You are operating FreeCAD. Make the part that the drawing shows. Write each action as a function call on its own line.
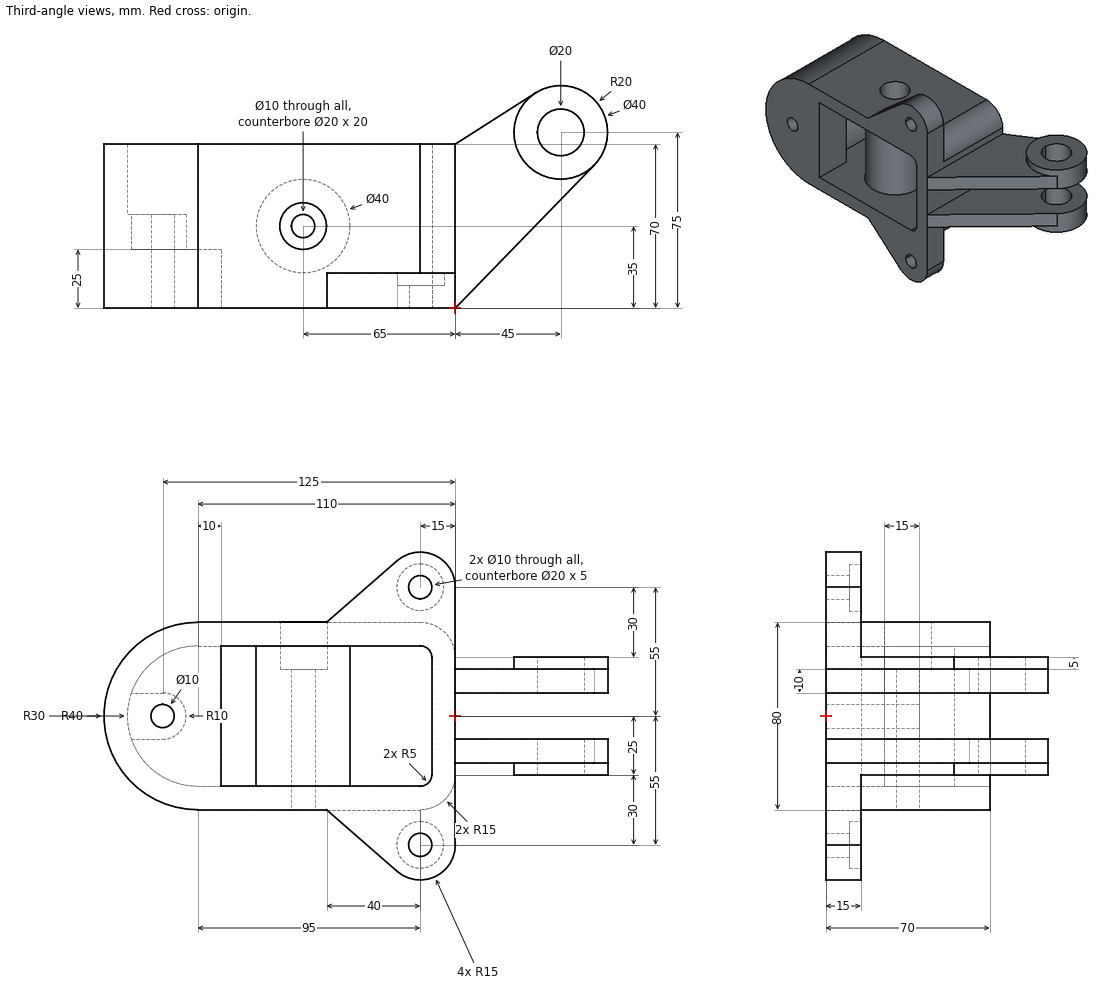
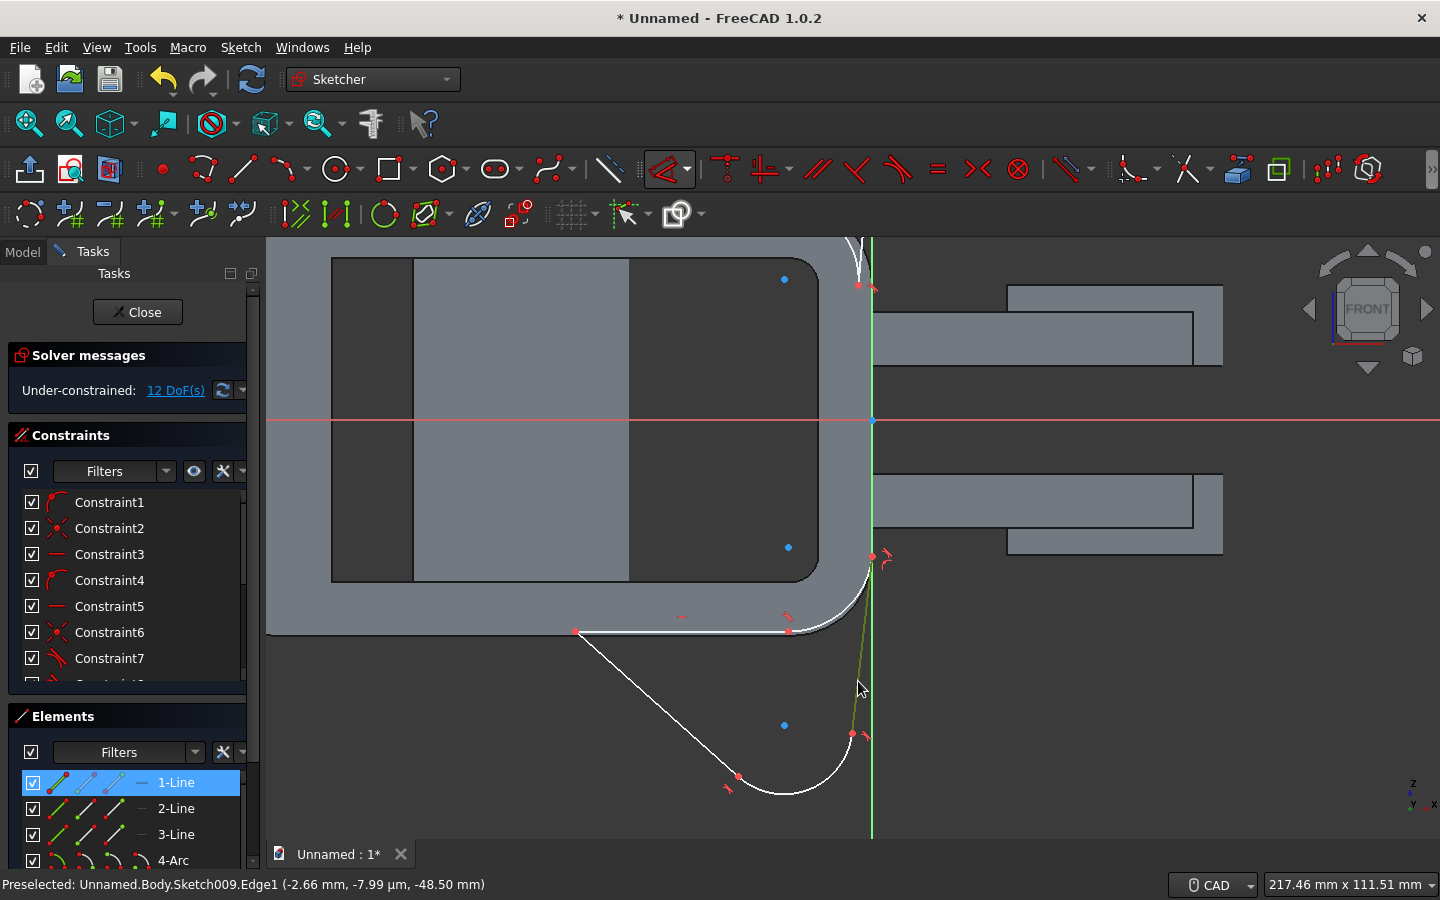
key(v)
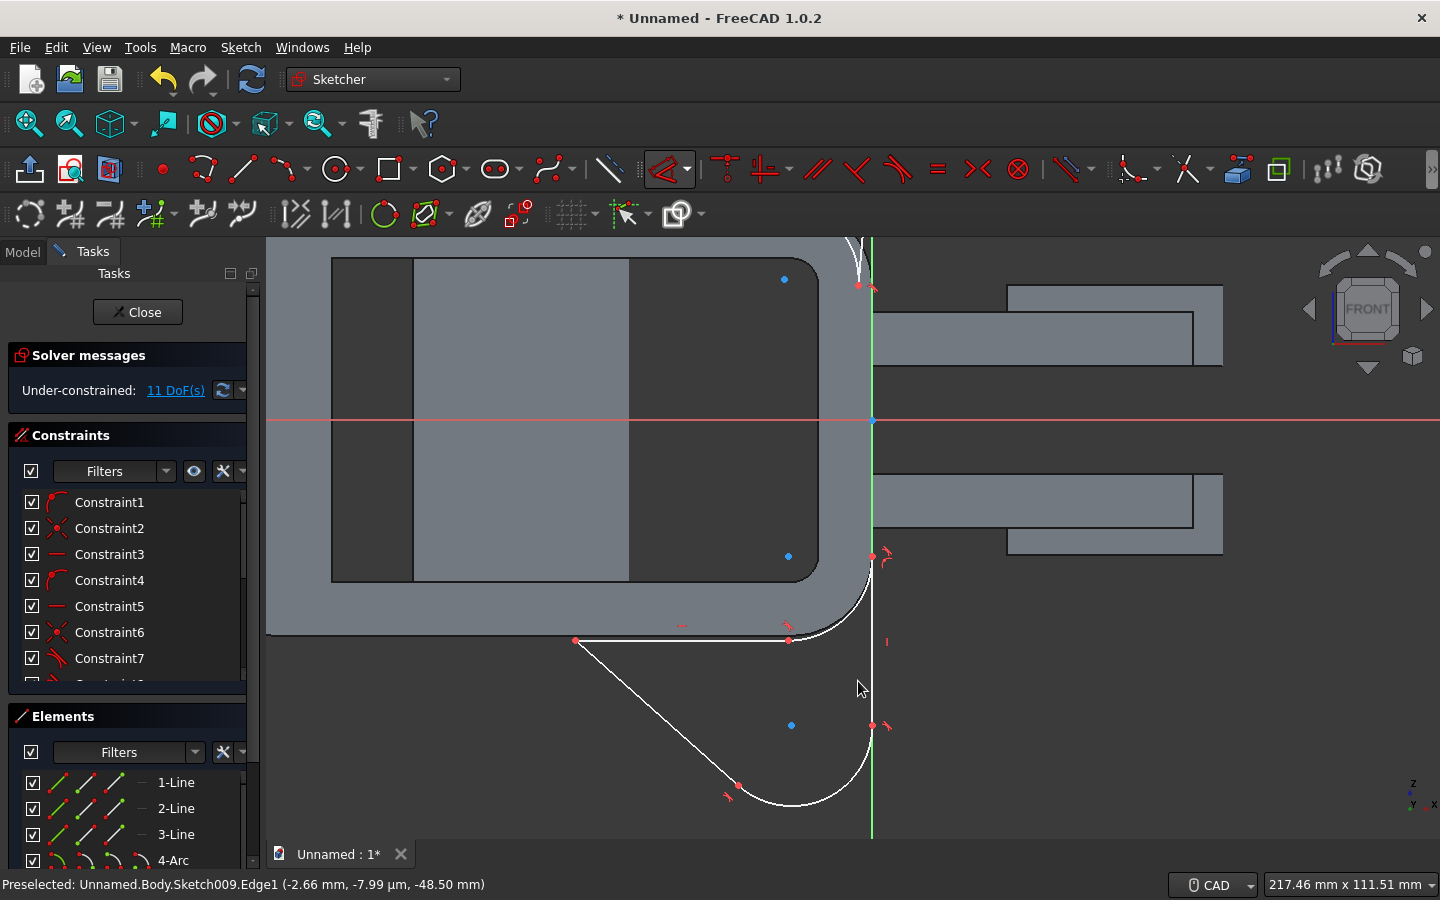
scroll(858, 681, down, 3)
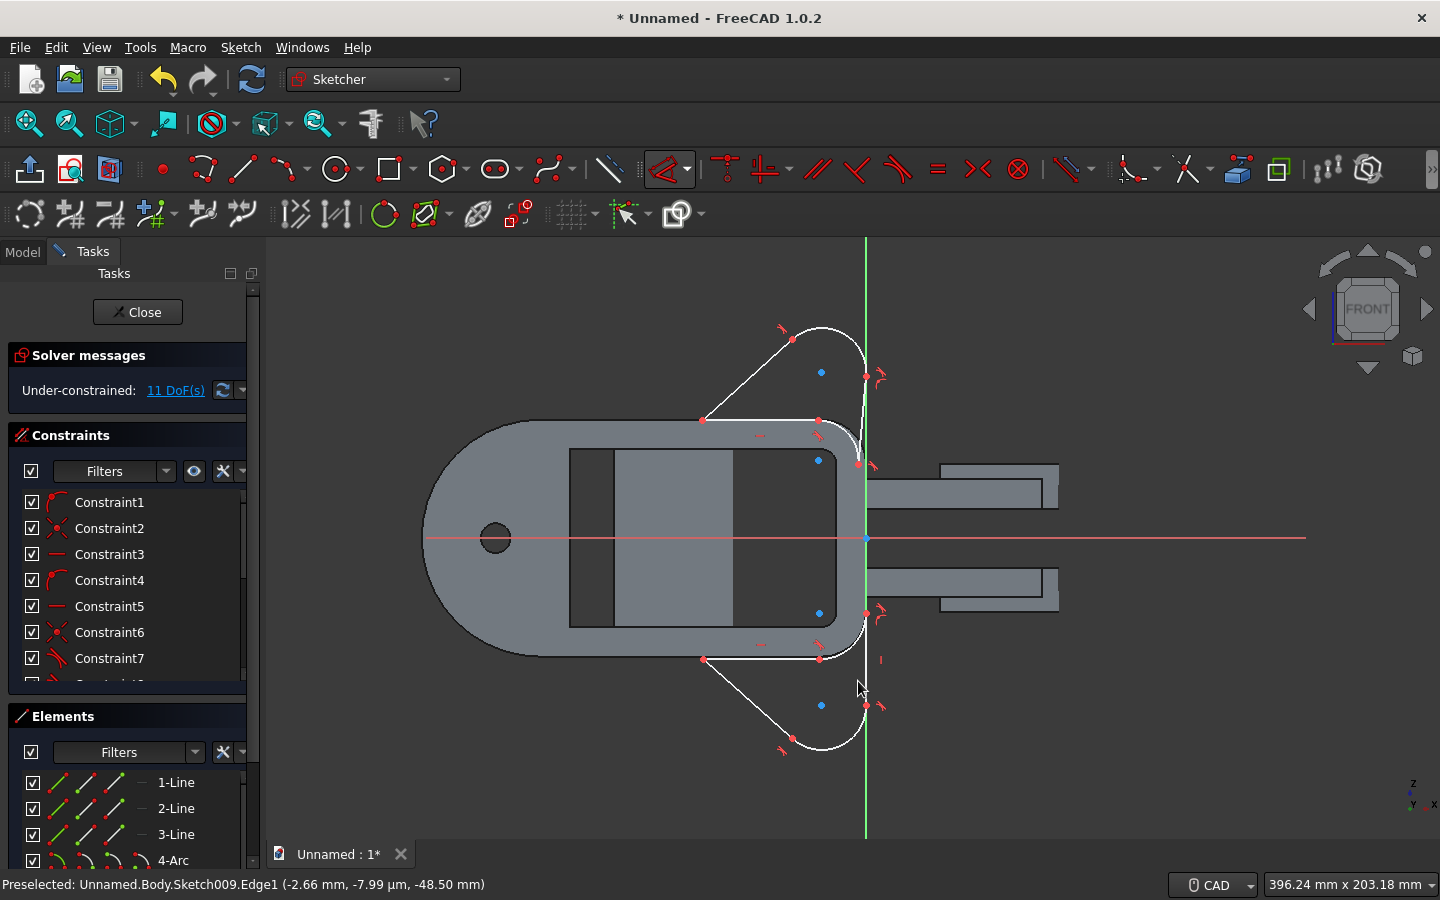
scroll(861, 438, up, 5)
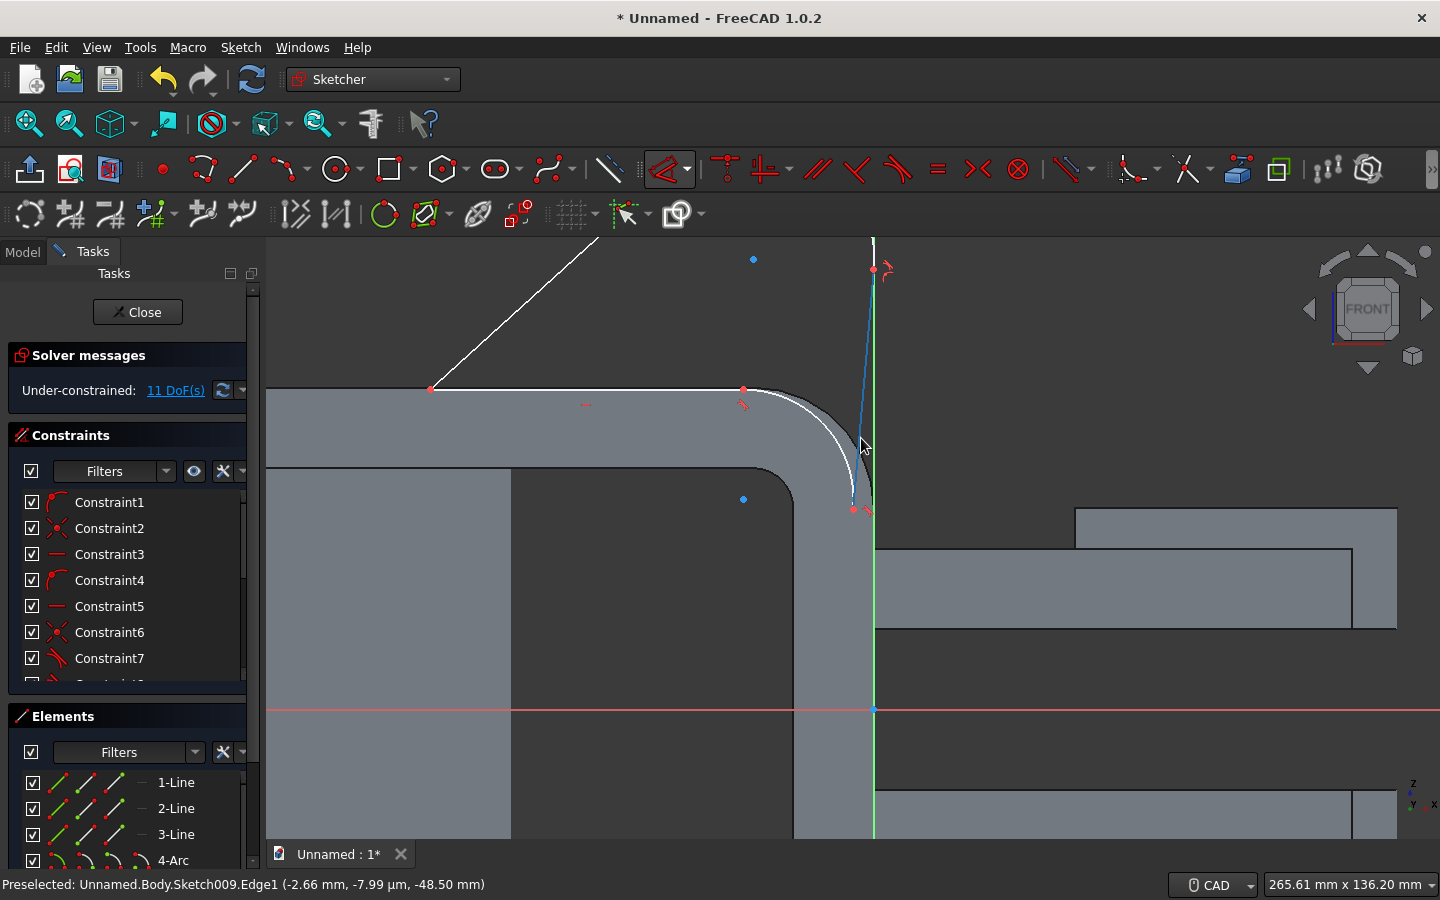
click(859, 437)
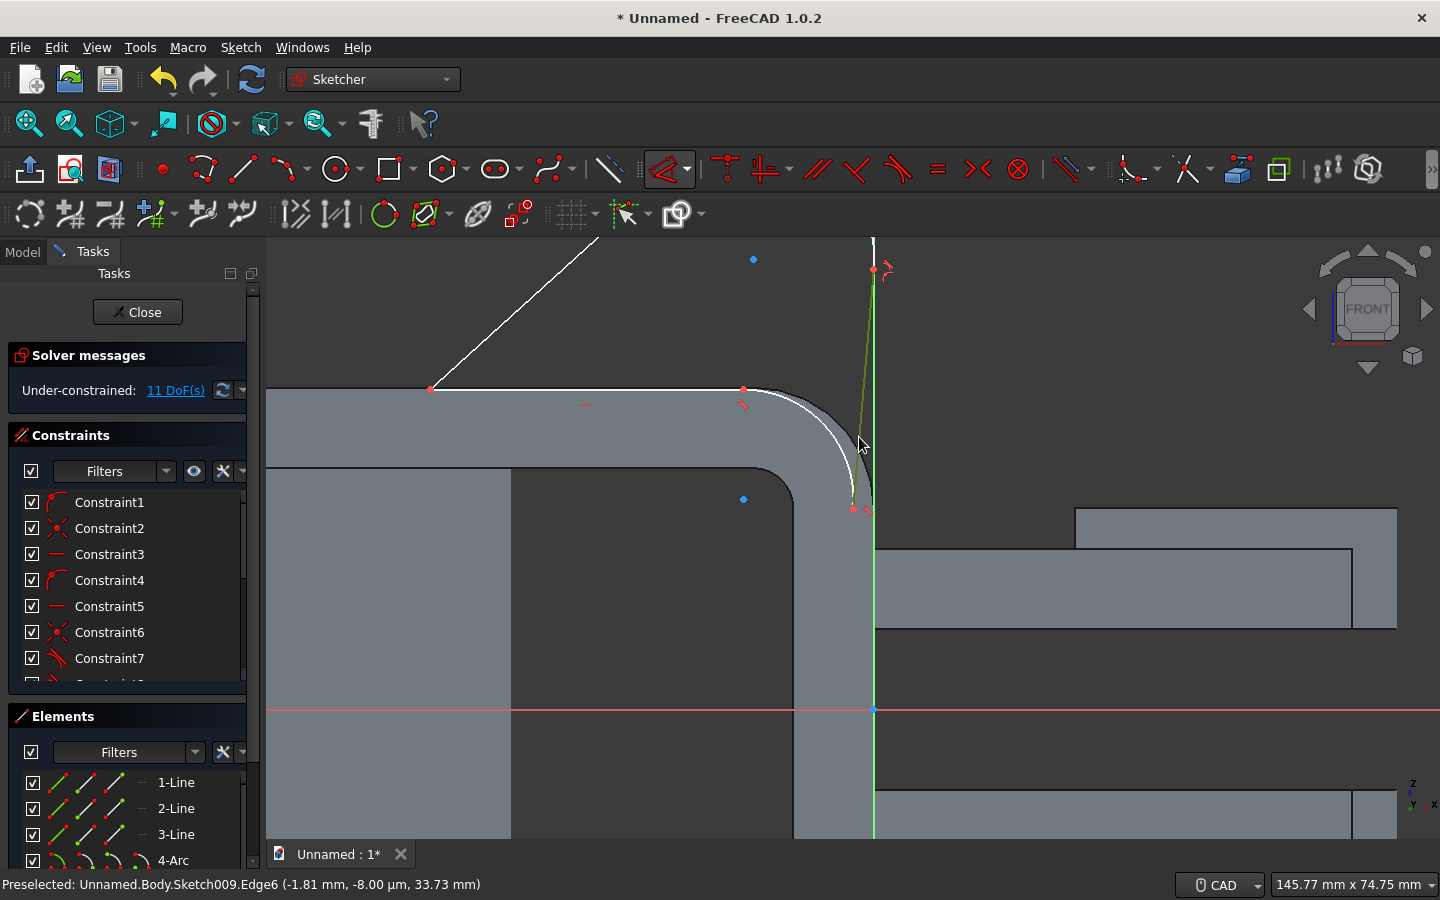
key(v)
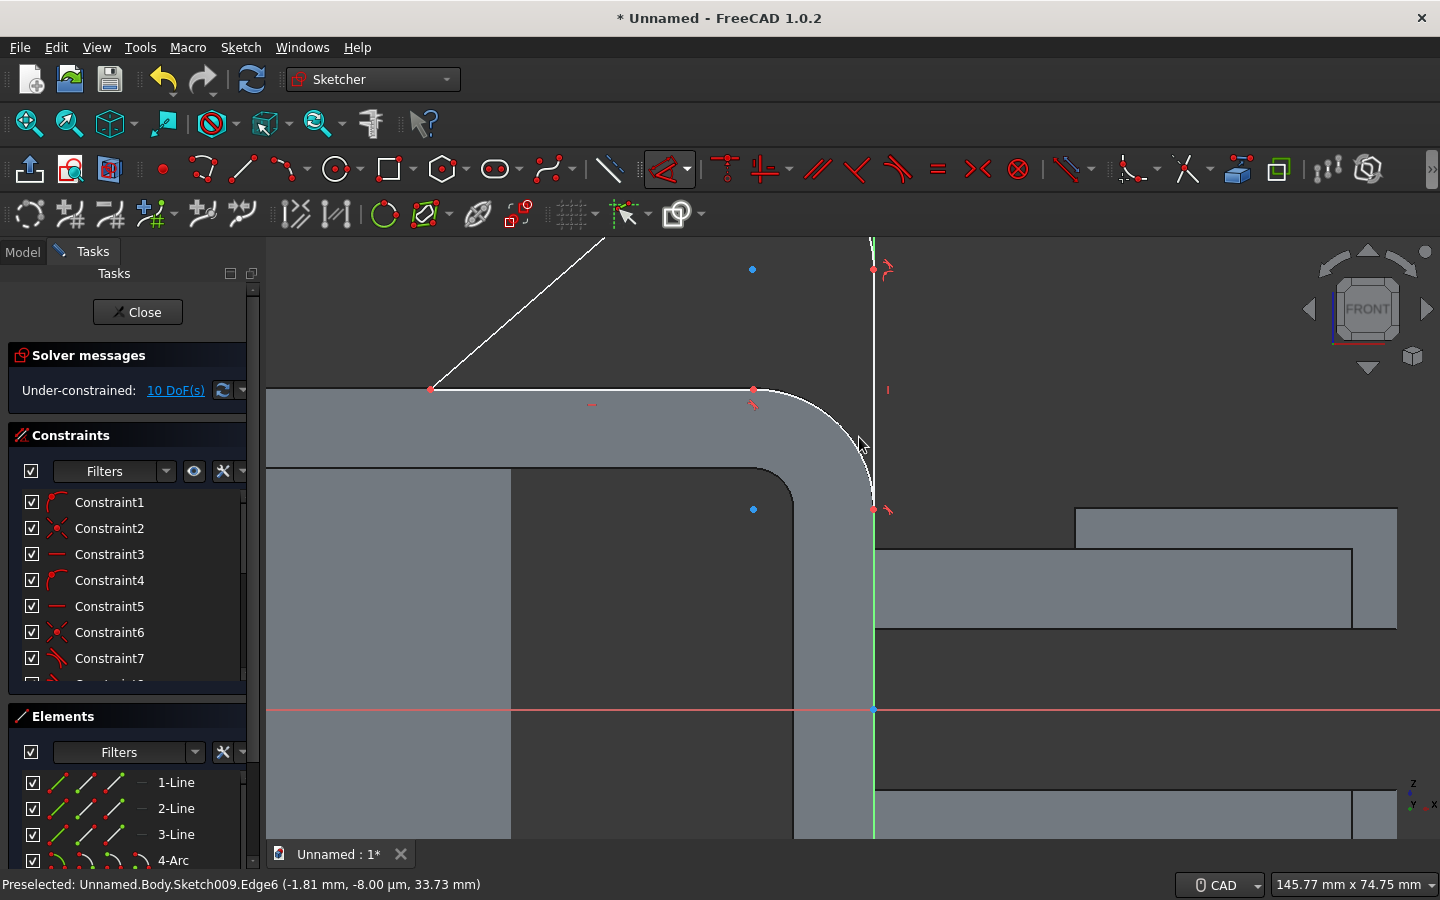
scroll(861, 438, down, 5)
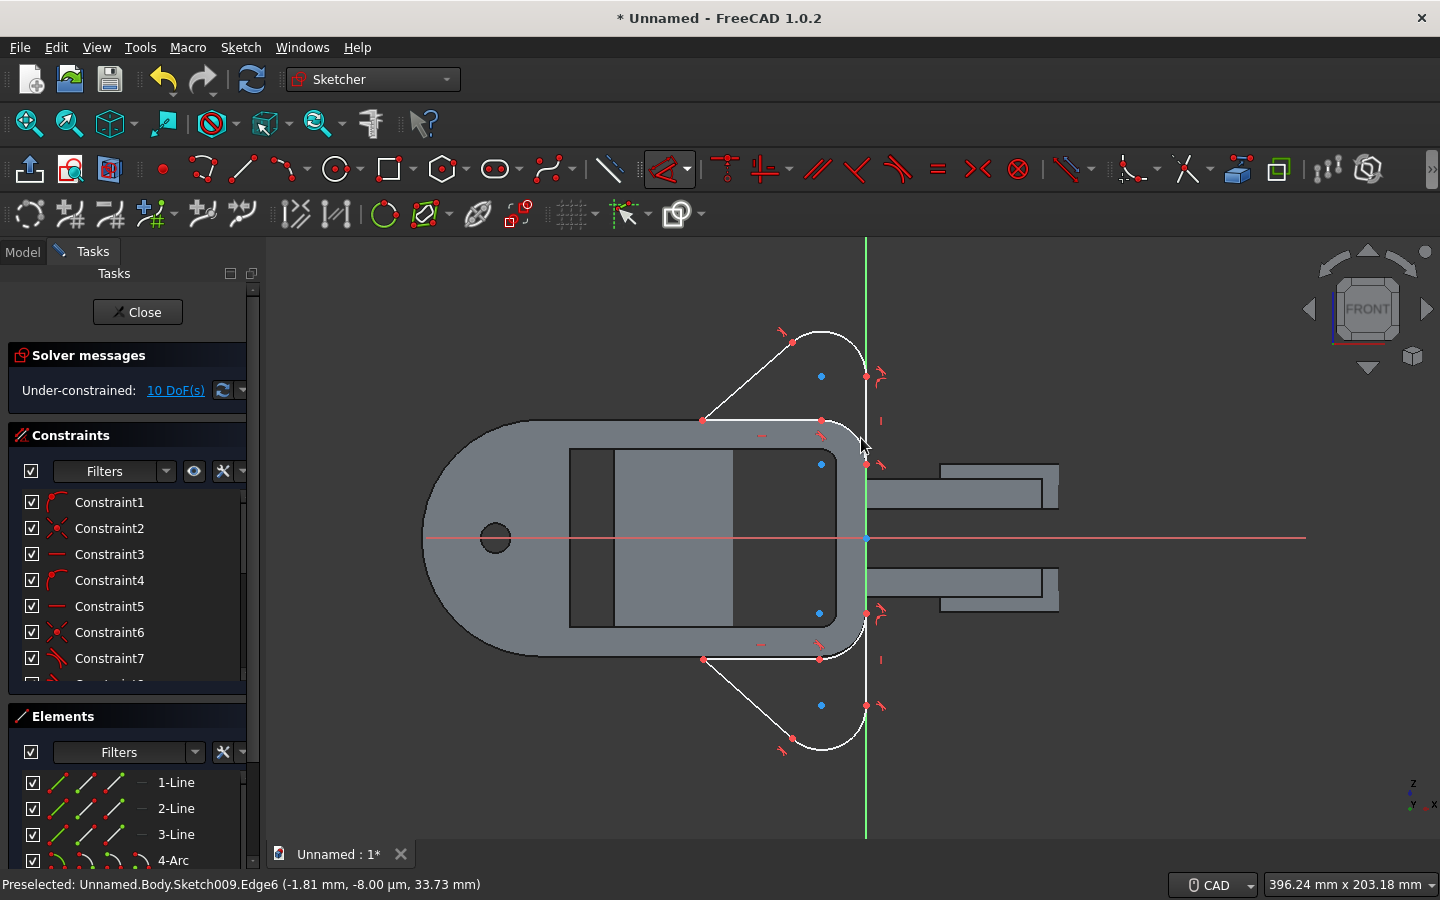
click(820, 750)